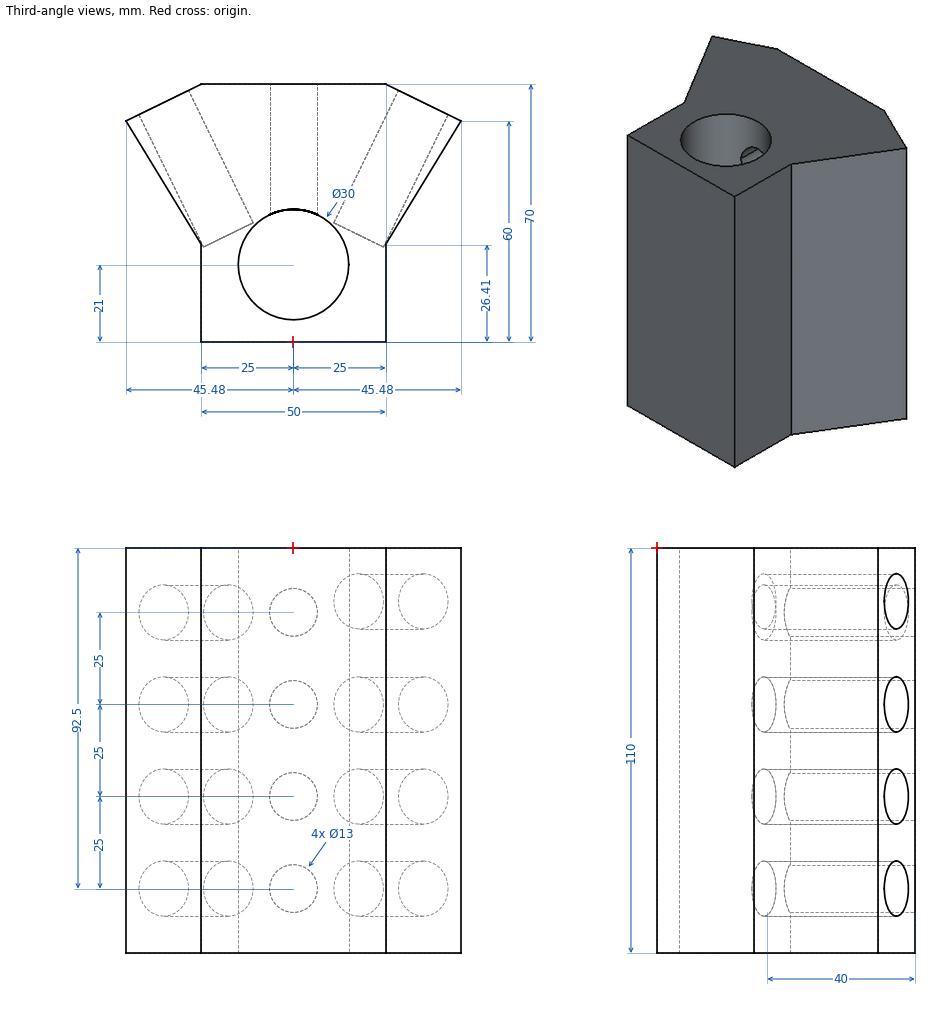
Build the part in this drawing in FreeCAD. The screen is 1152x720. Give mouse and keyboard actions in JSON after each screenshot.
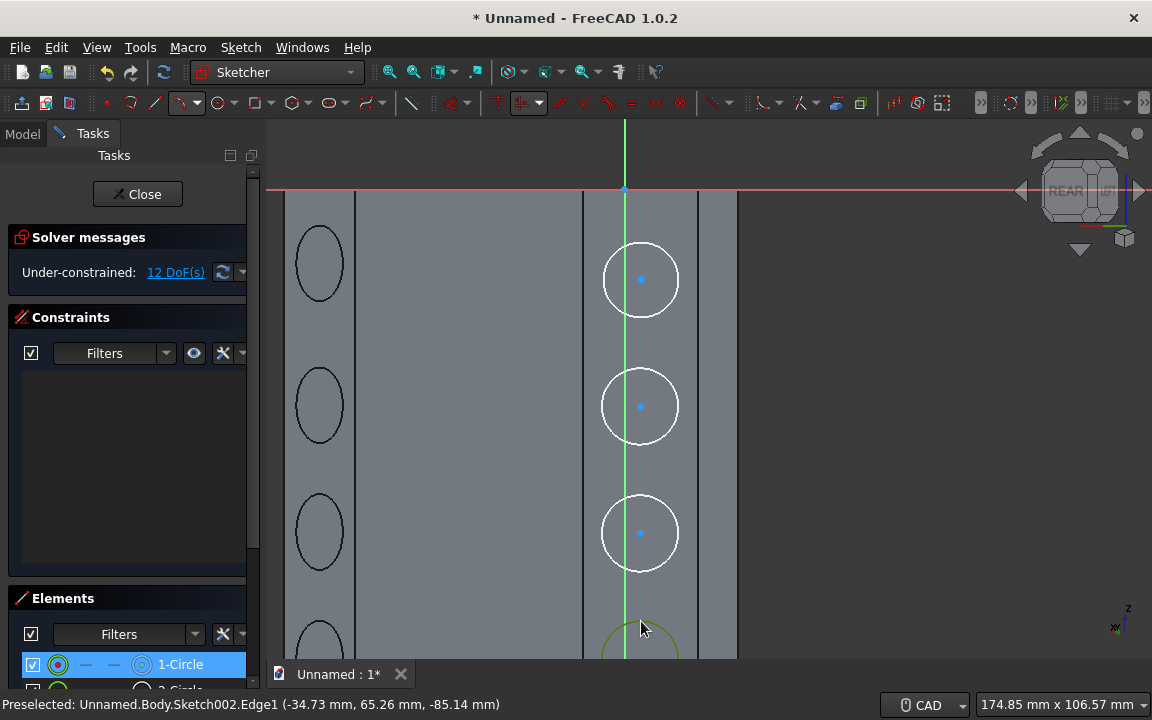
{"action": "left_click", "coordinate": [667, 506]}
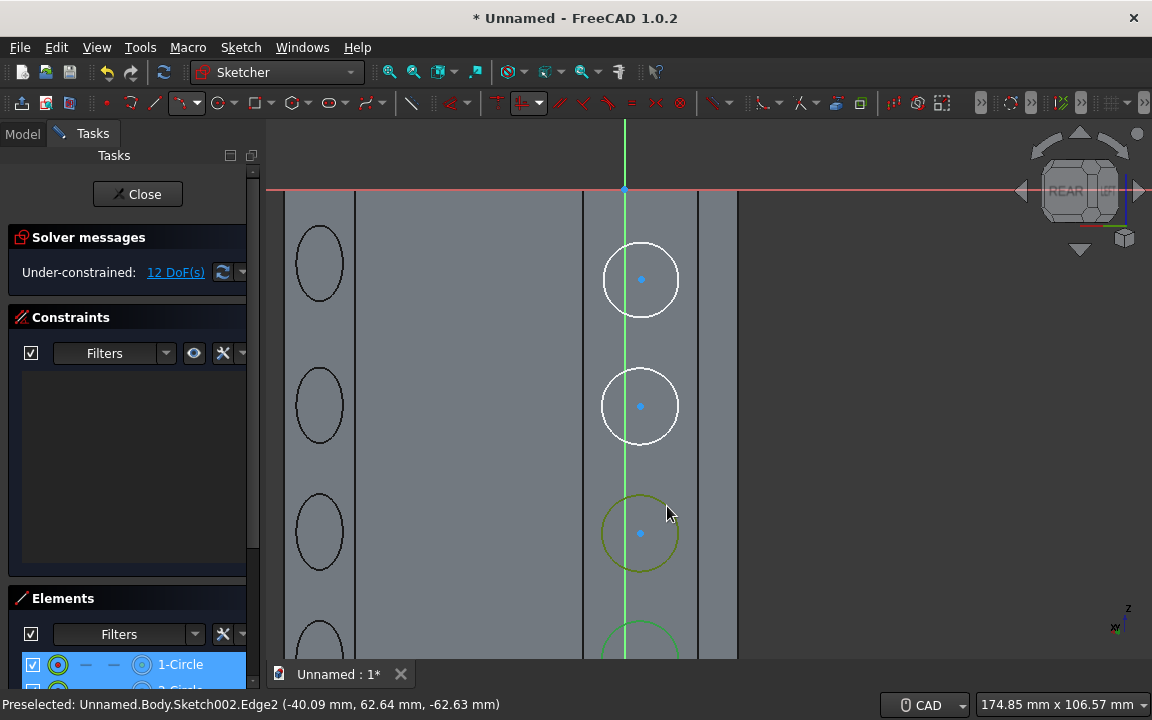
{"action": "left_click", "coordinate": [667, 379]}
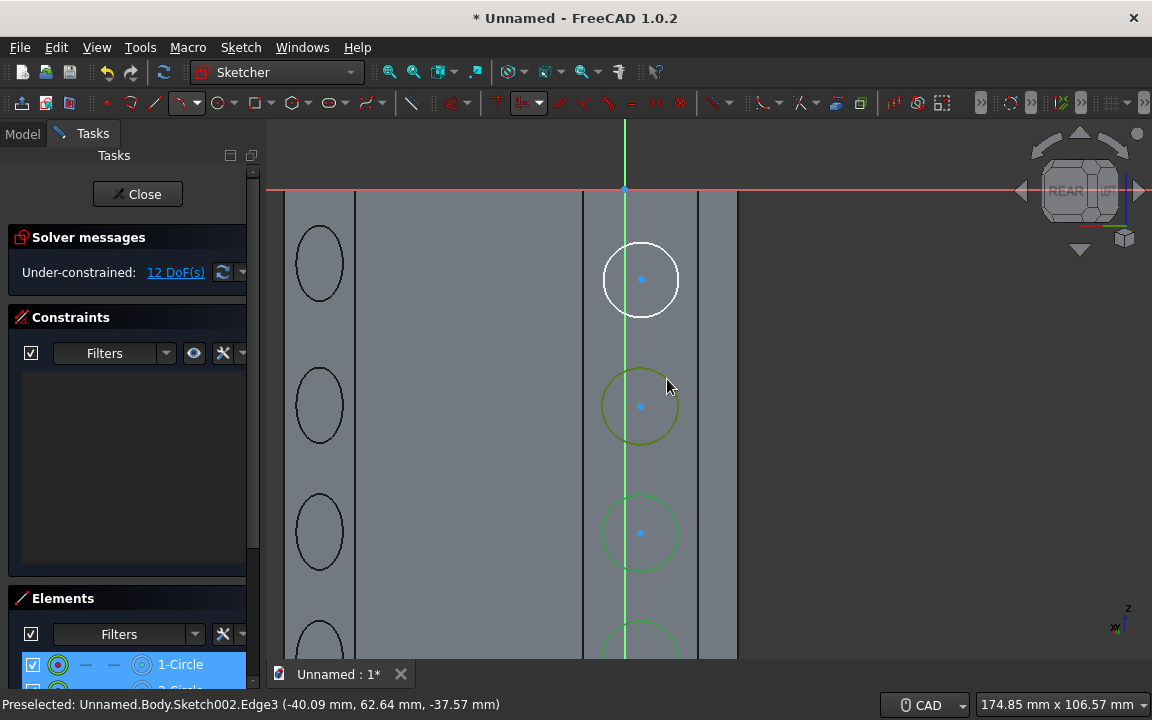
{"action": "left_click", "coordinate": [667, 253]}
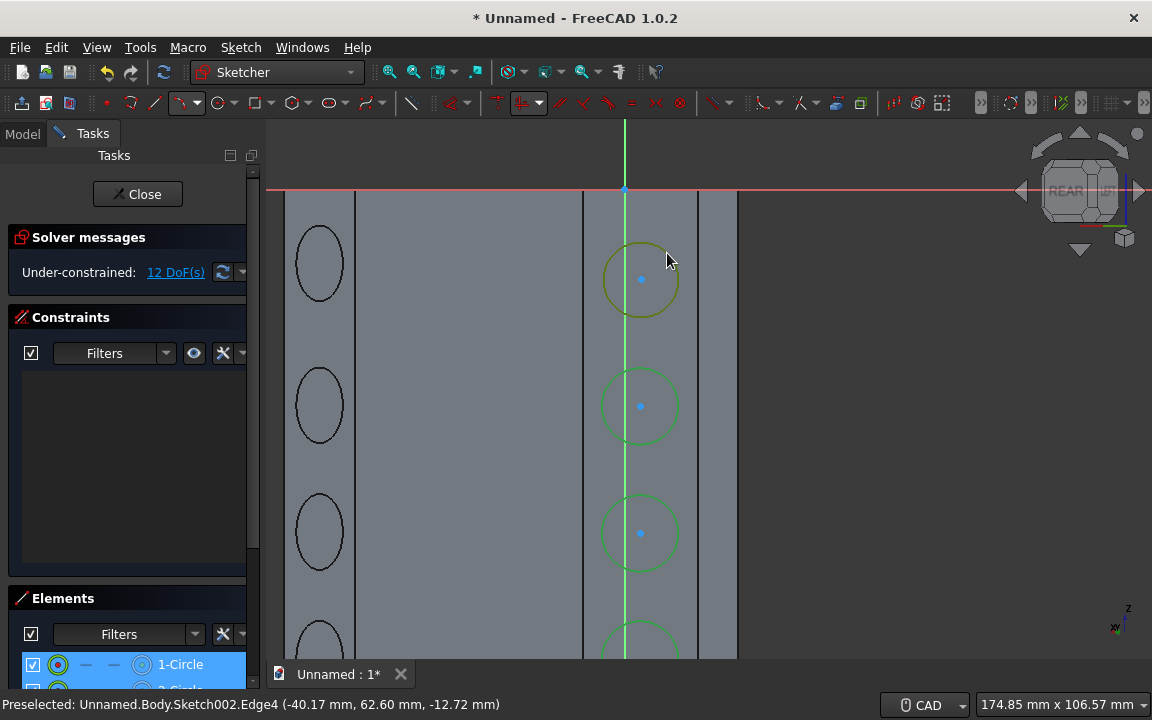
{"action": "left_click", "coordinate": [632, 104]}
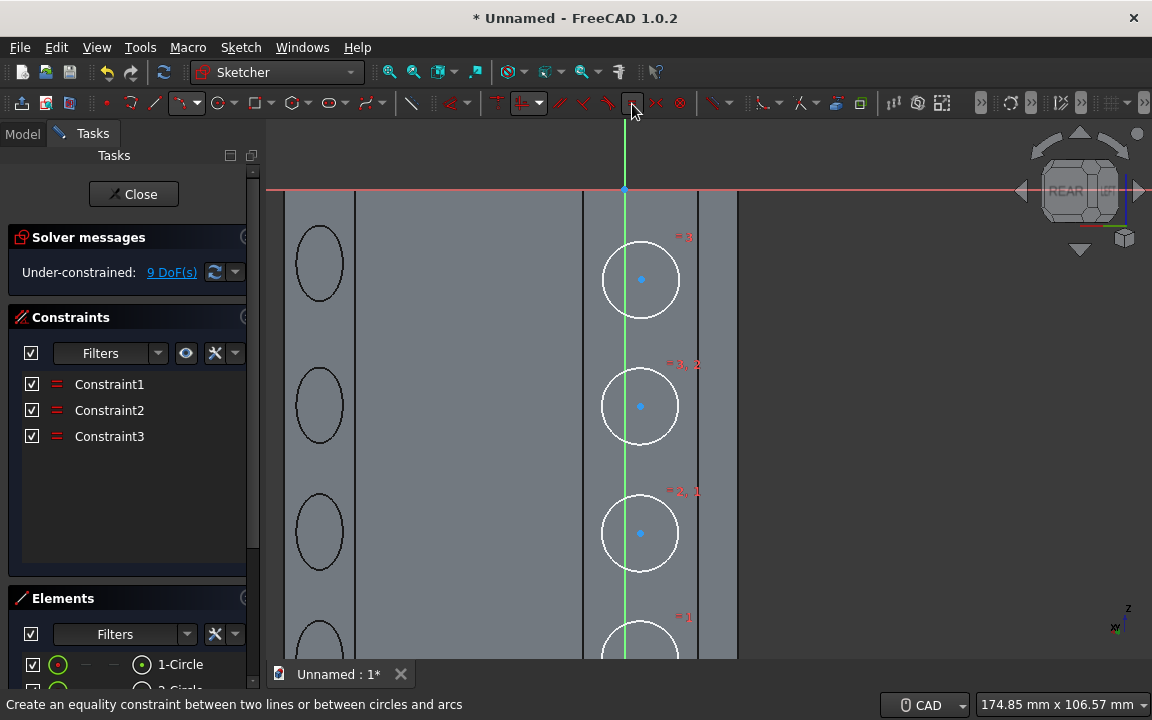
{"action": "left_click", "coordinate": [450, 104]}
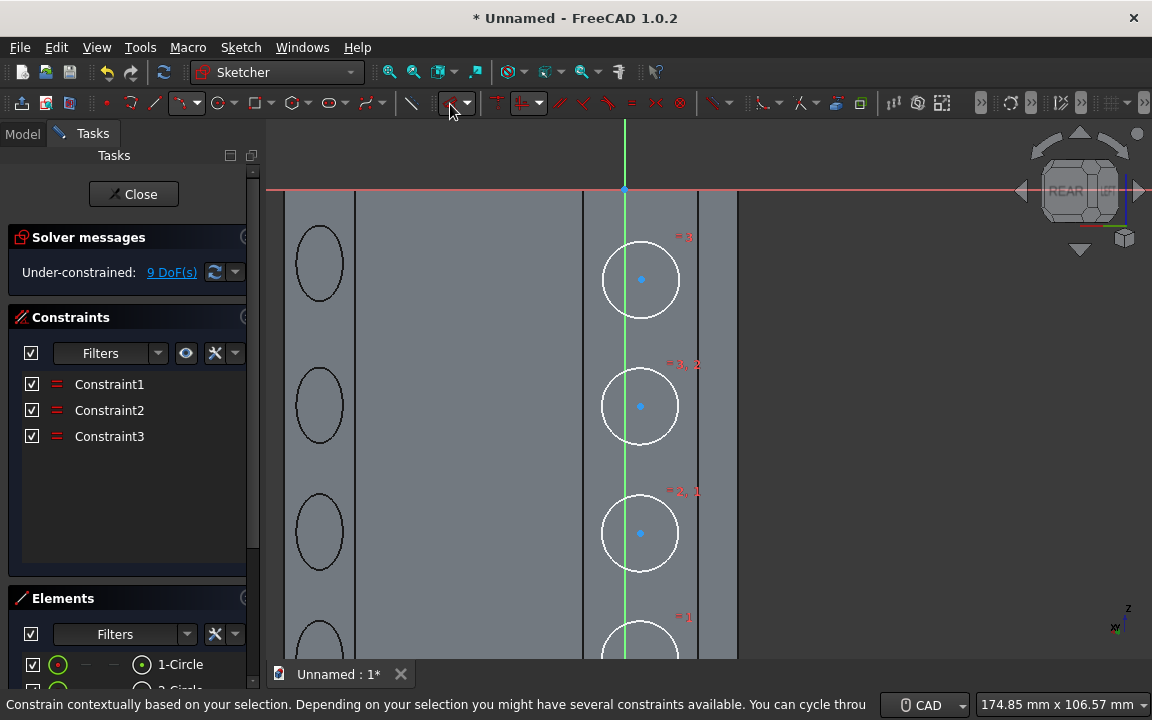
{"action": "left_click", "coordinate": [641, 621]}
{"action": "left_click", "coordinate": [642, 589]}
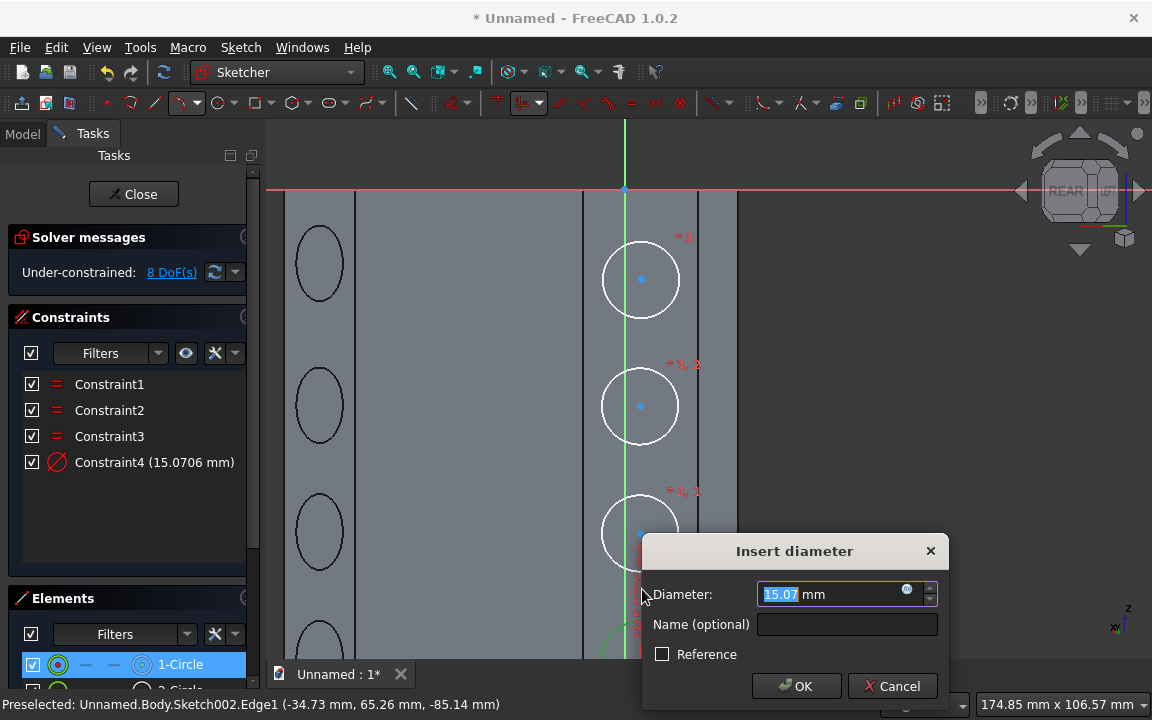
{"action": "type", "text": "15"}
{"action": "key", "text": "Return"}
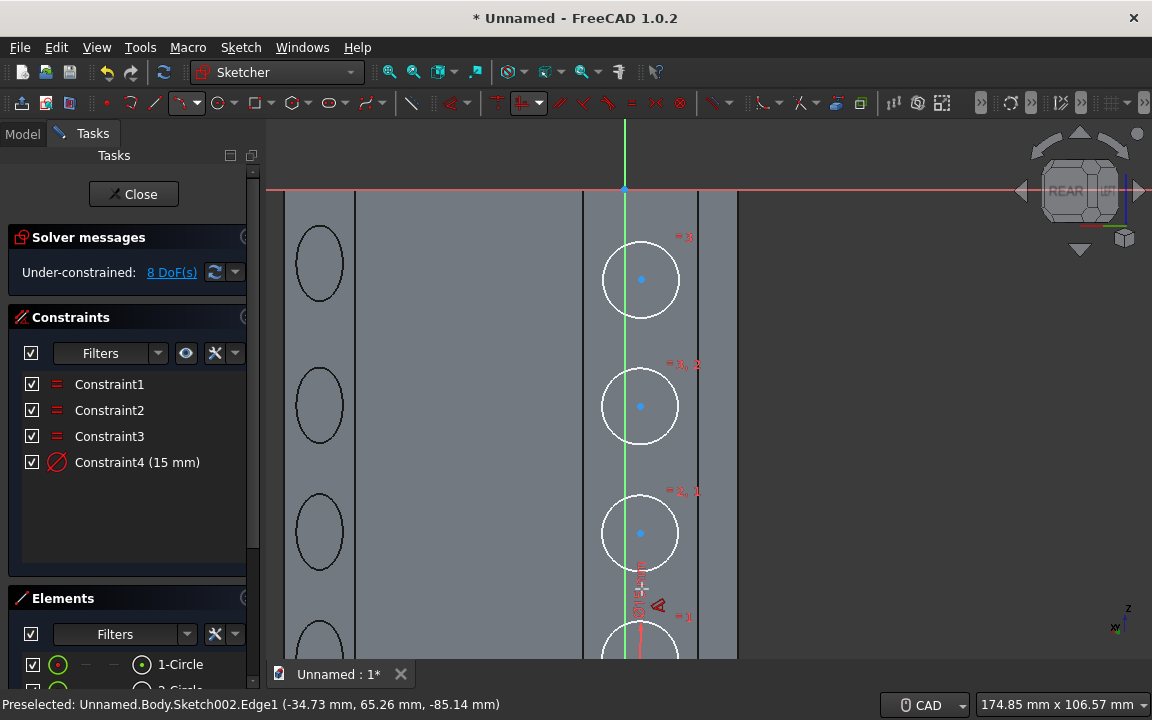
{"action": "scroll", "coordinate": [640, 279], "scroll_direction": "down", "scroll_amount": 2}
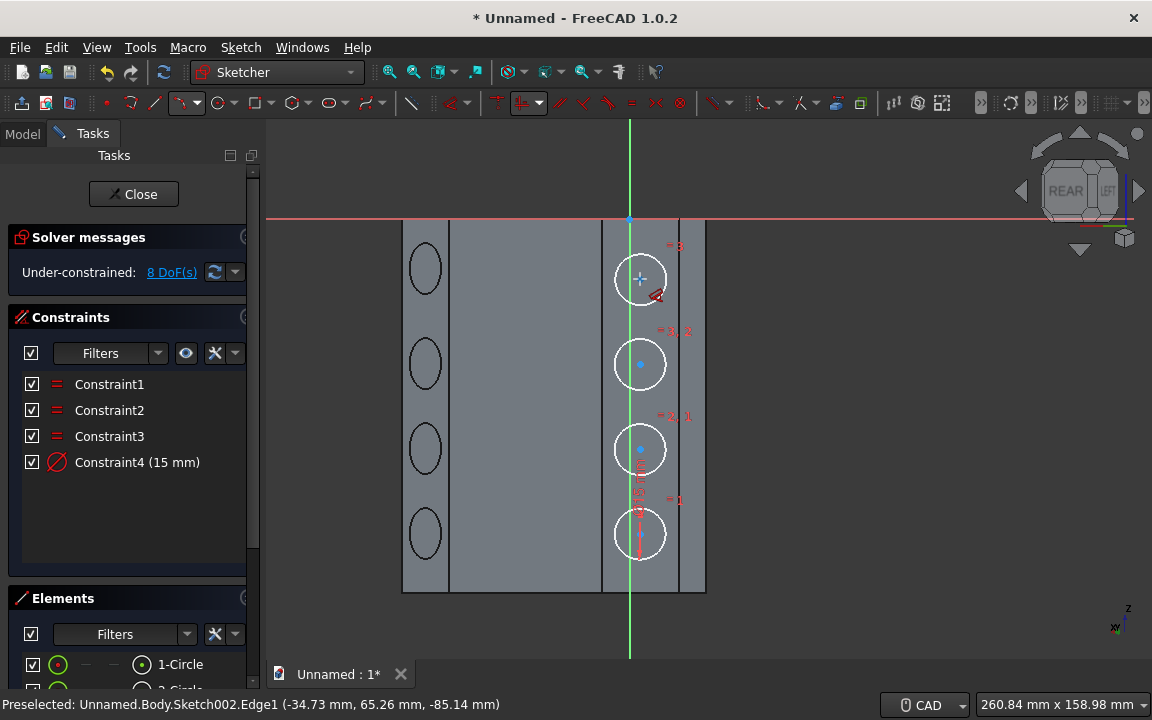
{"action": "left_click", "coordinate": [640, 534]}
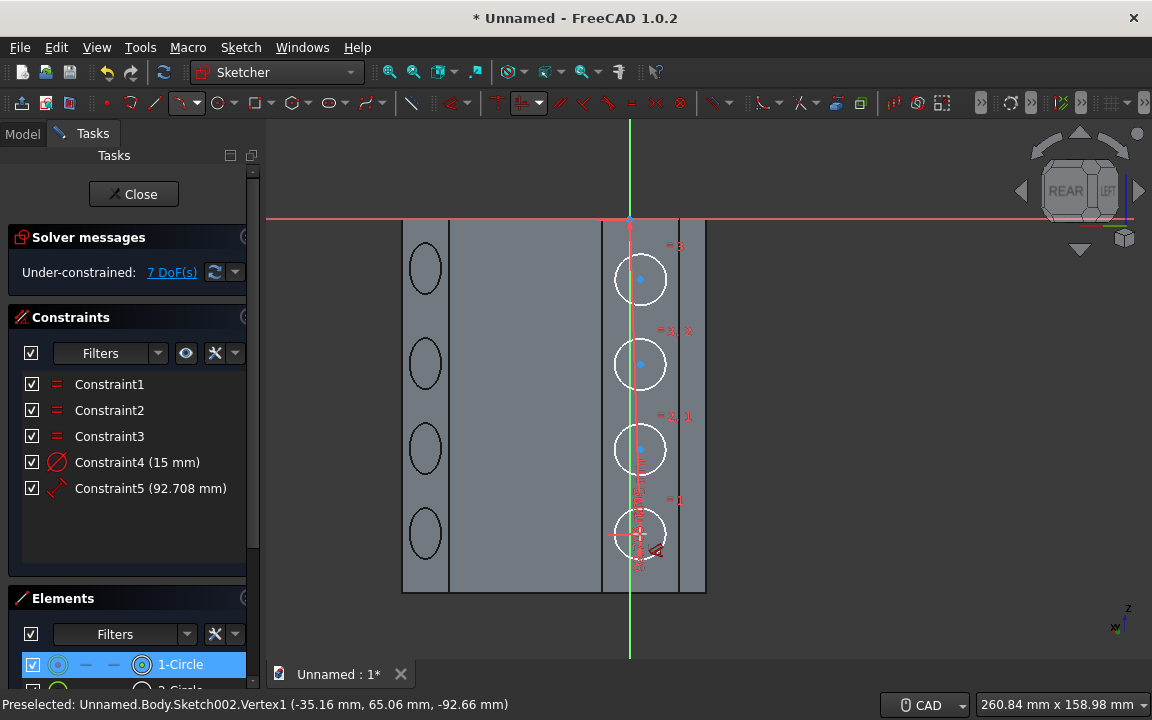
{"action": "left_click", "coordinate": [640, 450]}
{"action": "left_click", "coordinate": [606, 511]}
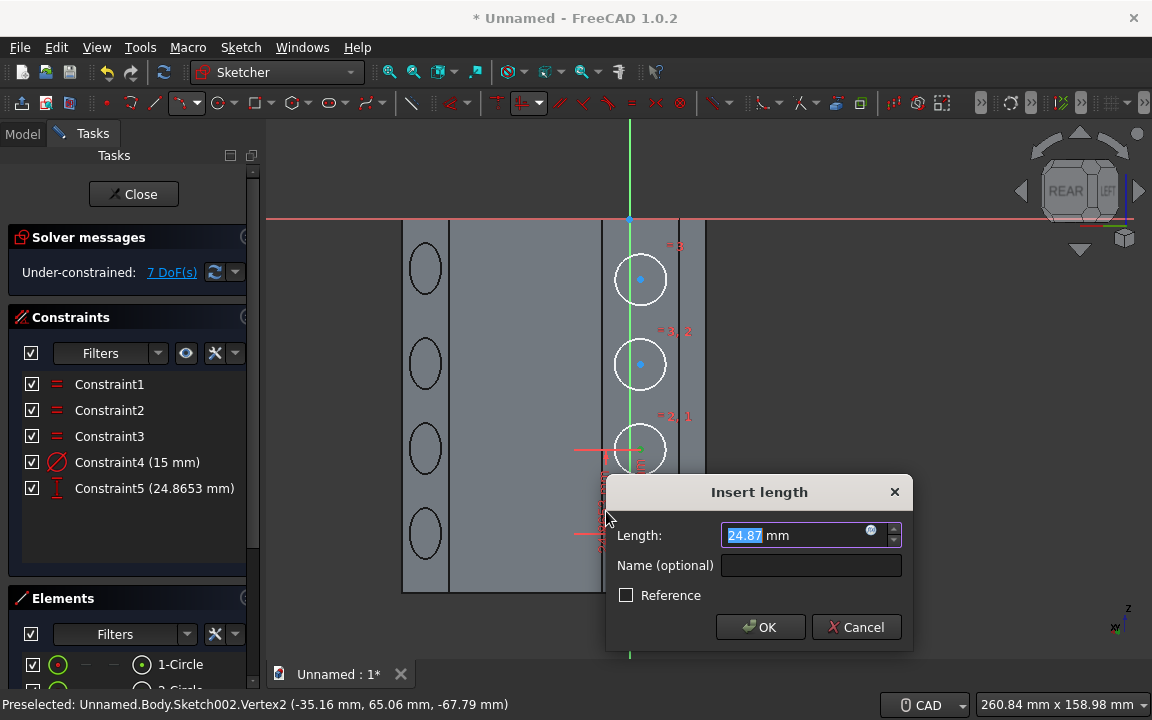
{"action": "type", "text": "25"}
{"action": "key", "text": "Return"}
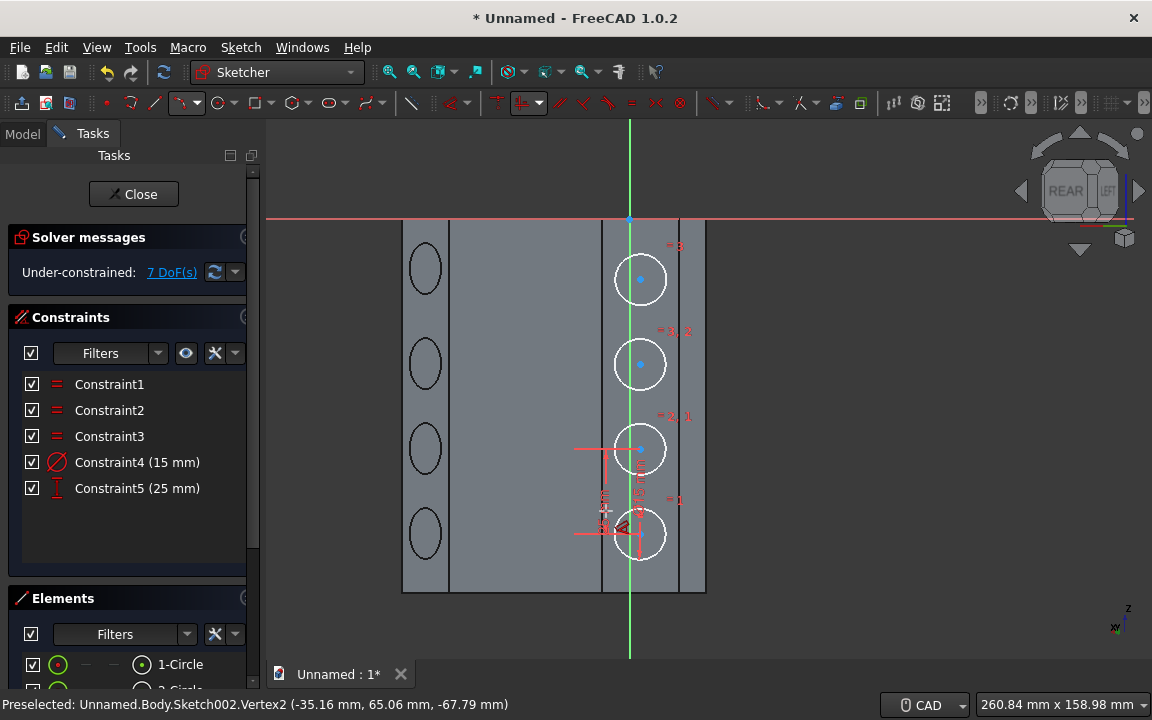
{"action": "left_click", "coordinate": [640, 449]}